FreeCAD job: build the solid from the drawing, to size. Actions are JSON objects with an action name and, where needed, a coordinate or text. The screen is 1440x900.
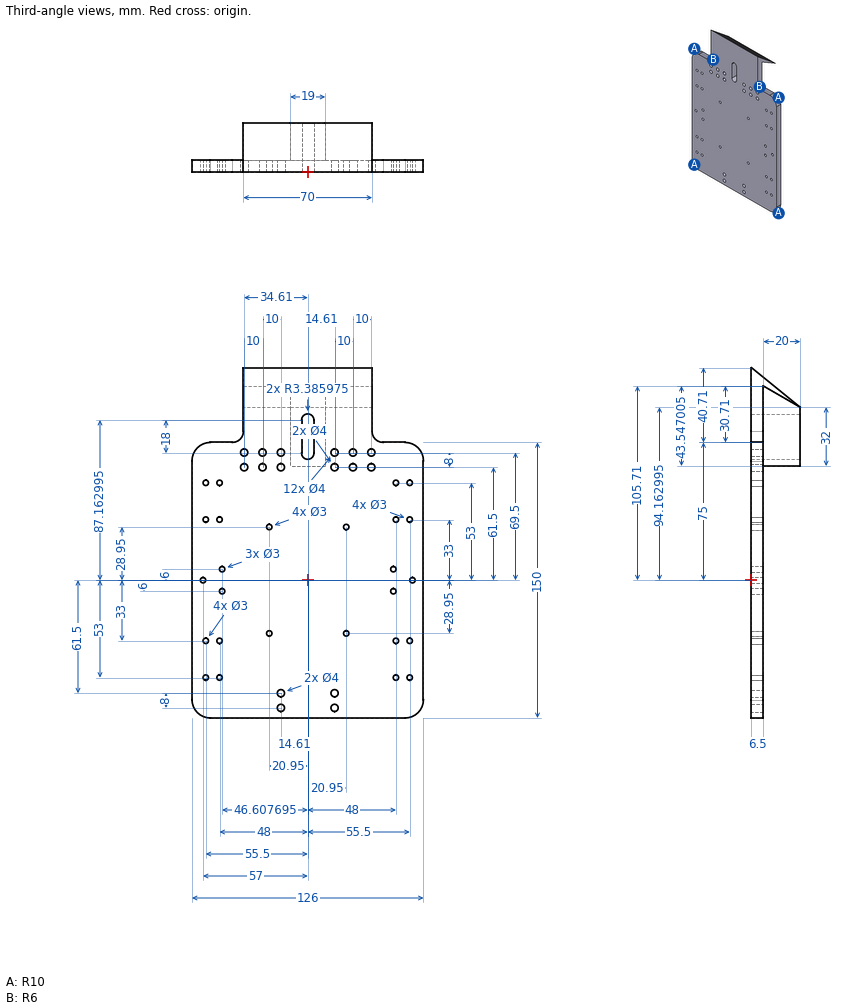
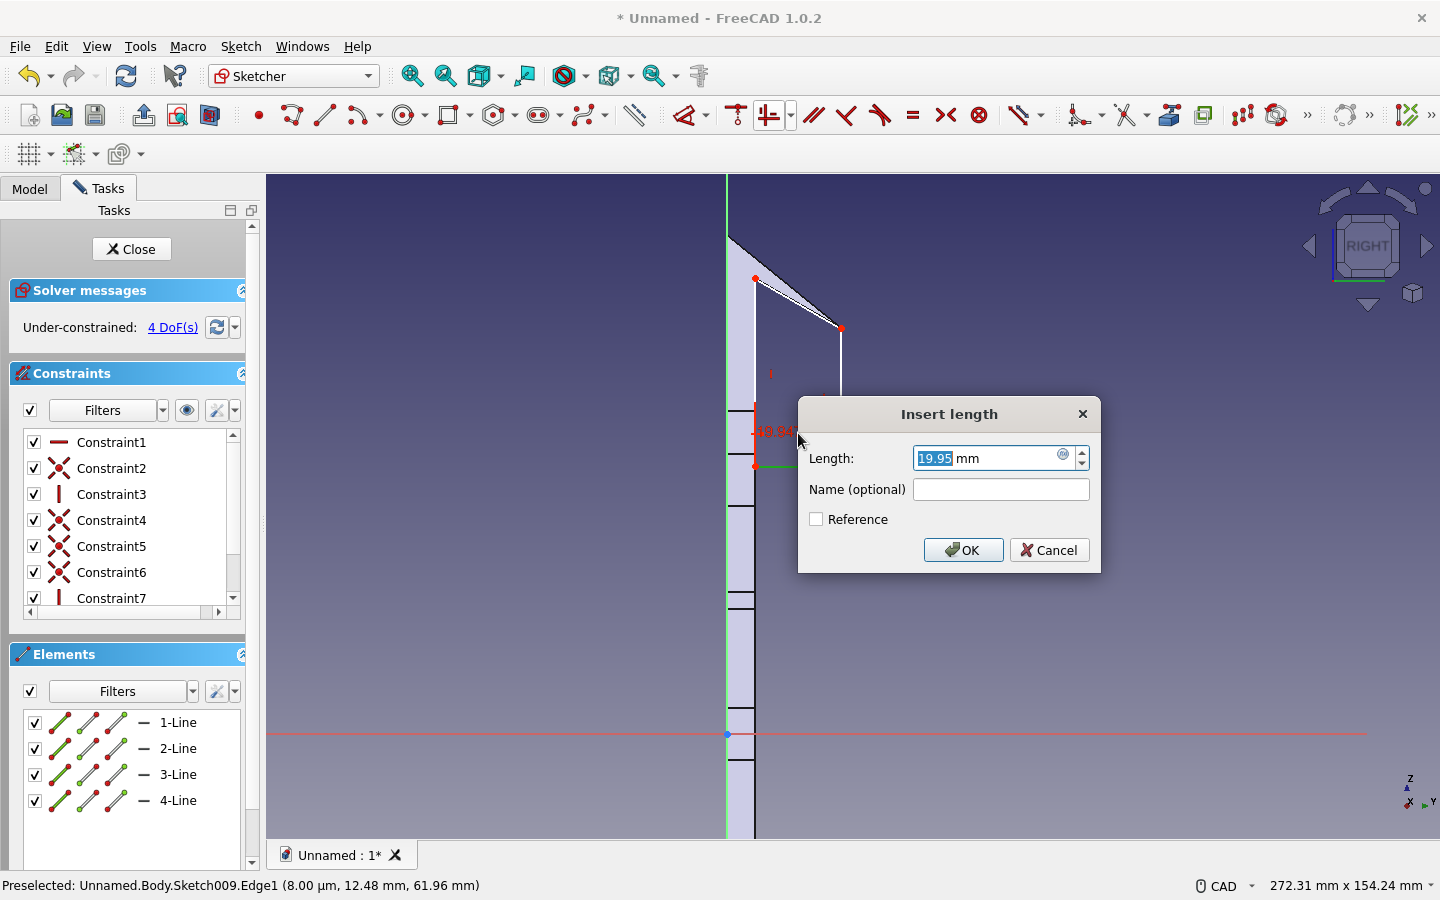
{"action": "type", "text": "20"}
{"action": "key", "text": "Return"}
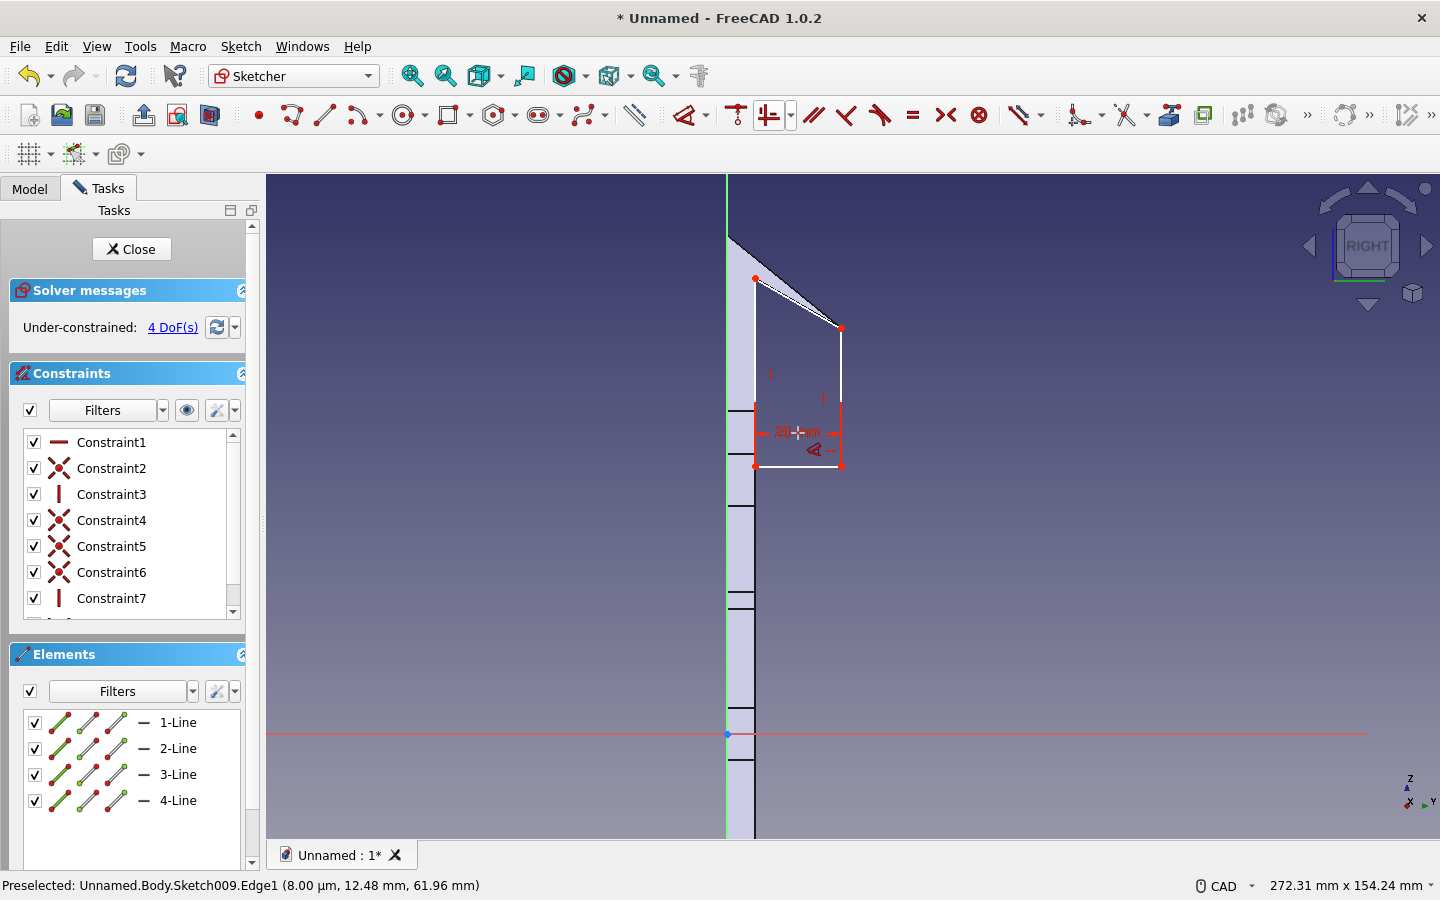
{"action": "left_click", "coordinate": [841, 426]}
{"action": "left_click", "coordinate": [875, 398]}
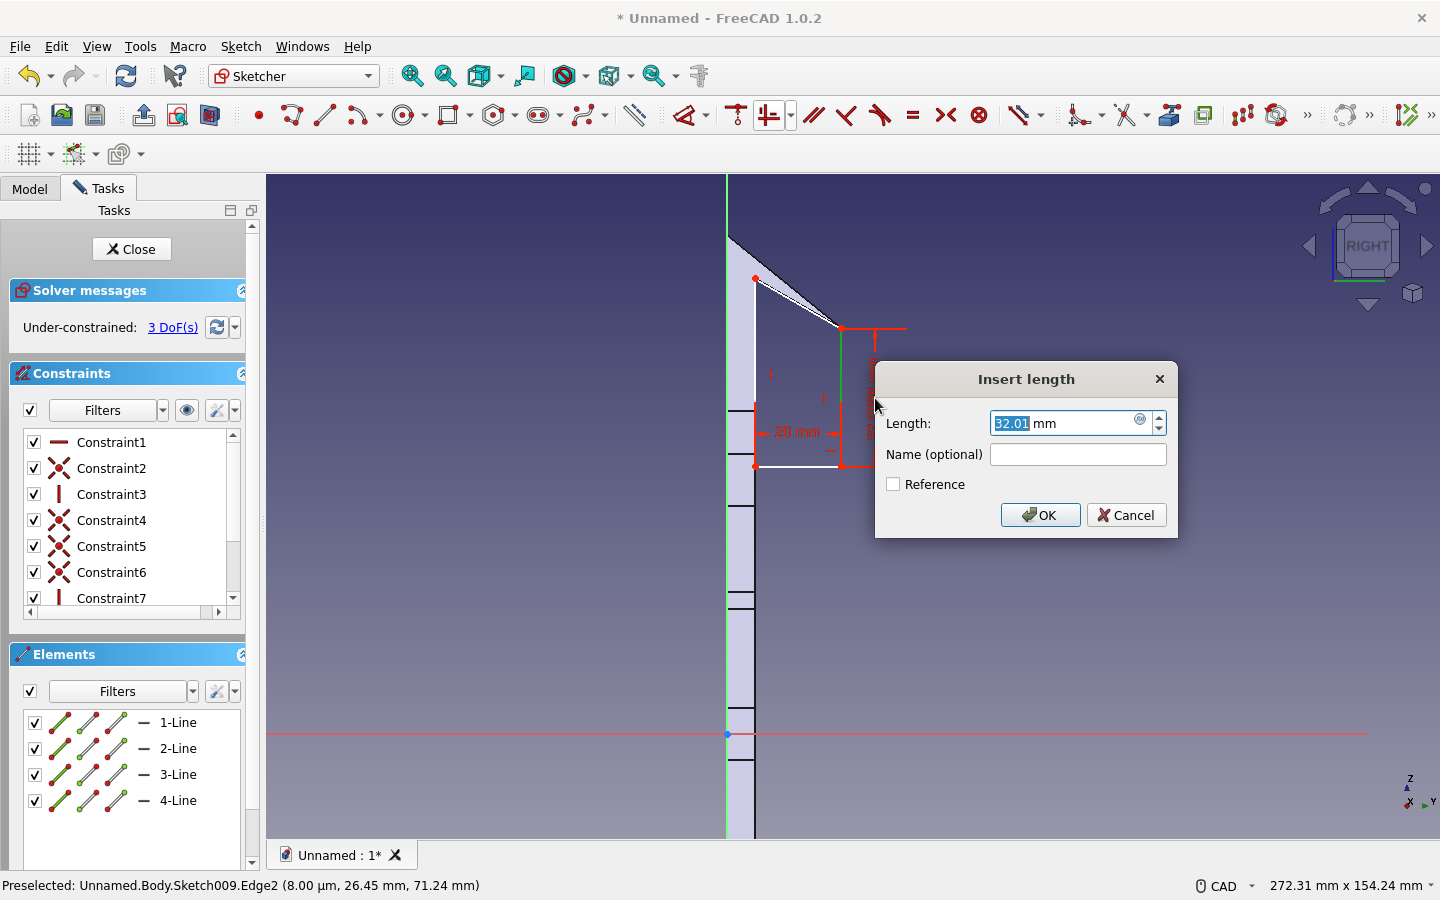
{"action": "type", "text": "32"}
{"action": "key", "text": "Return"}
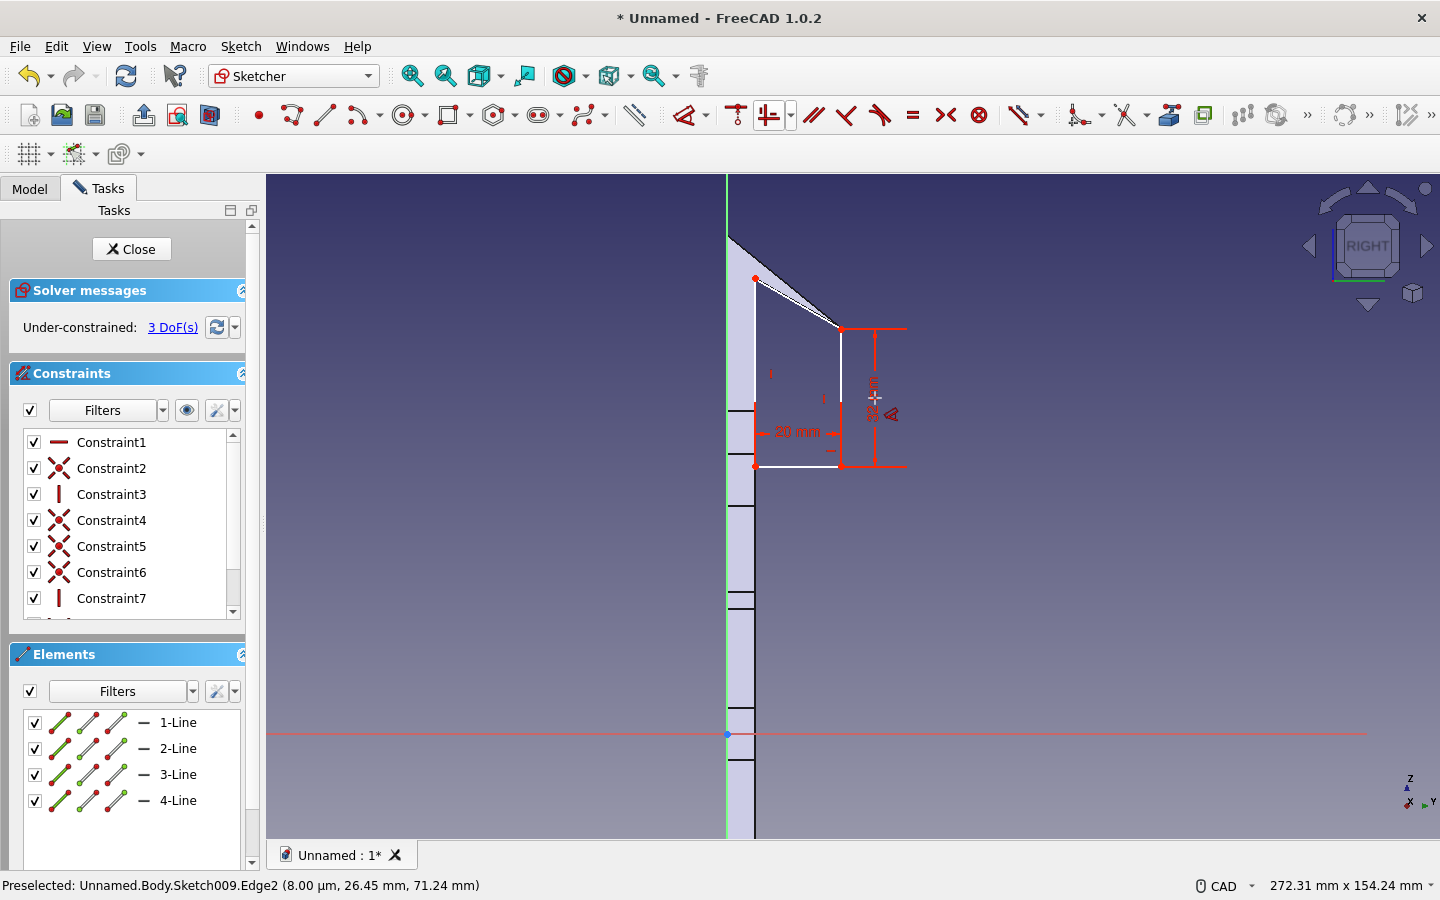
{"action": "scroll", "coordinate": [755, 467], "scroll_direction": "up", "scroll_amount": 2}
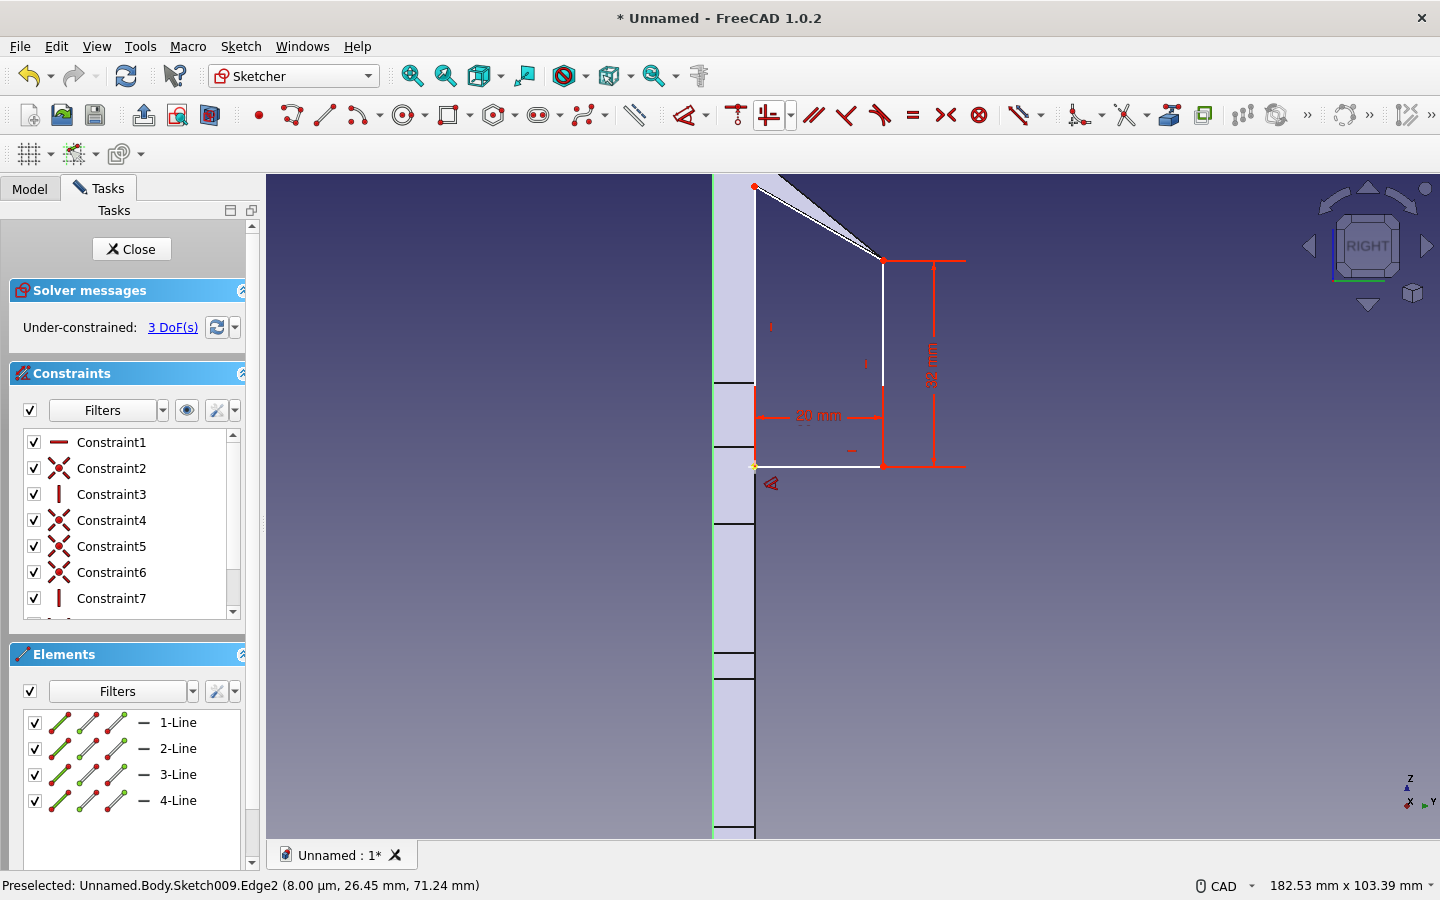
{"action": "left_click", "coordinate": [755, 467]}
{"action": "left_click", "coordinate": [734, 433]}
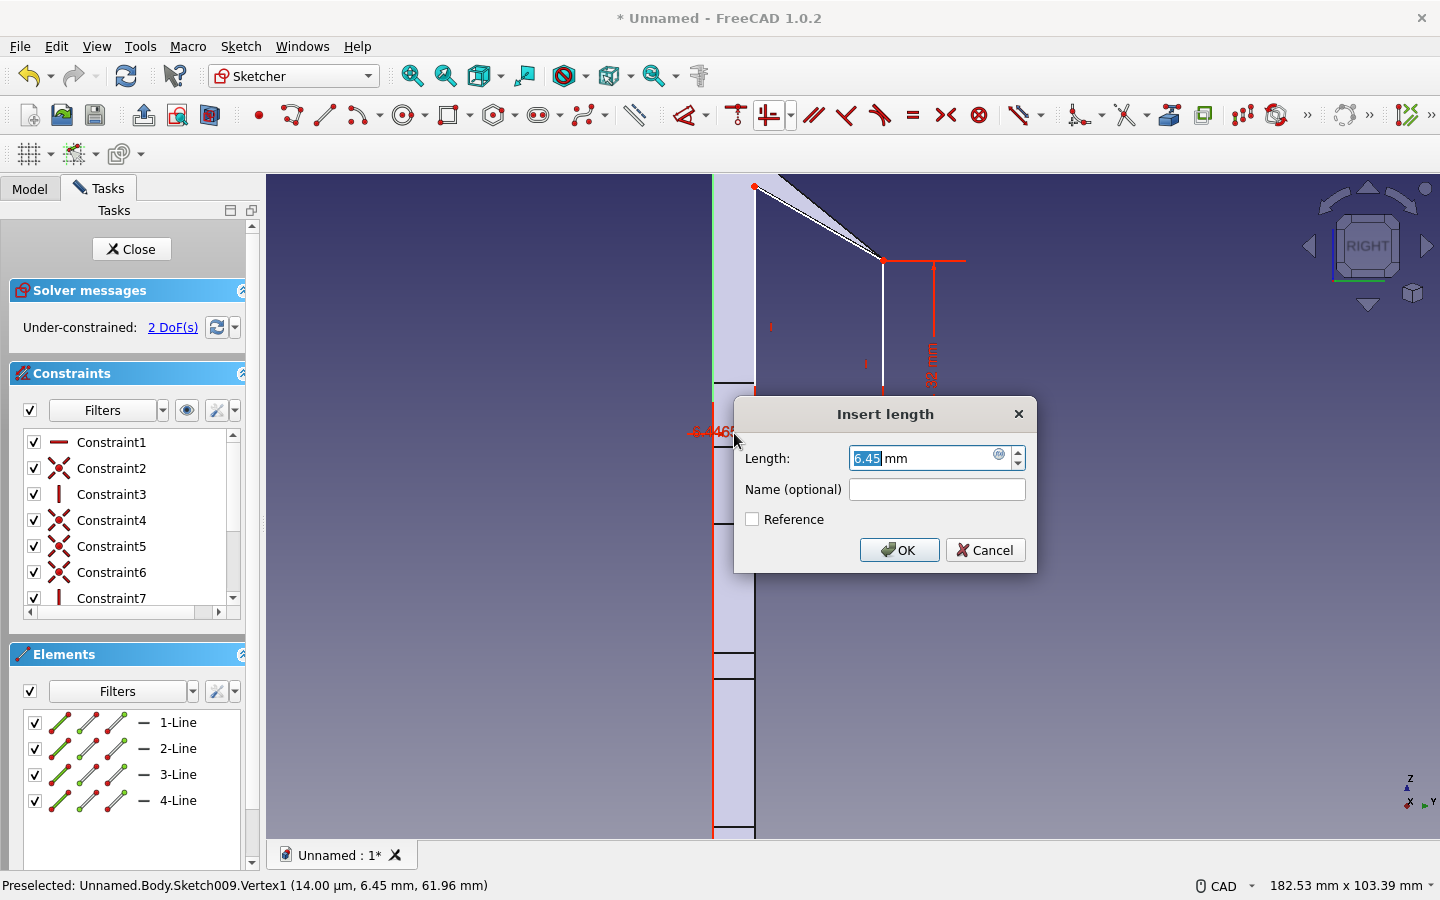
{"action": "type", "text": "6.5"}
{"action": "key", "text": "Return"}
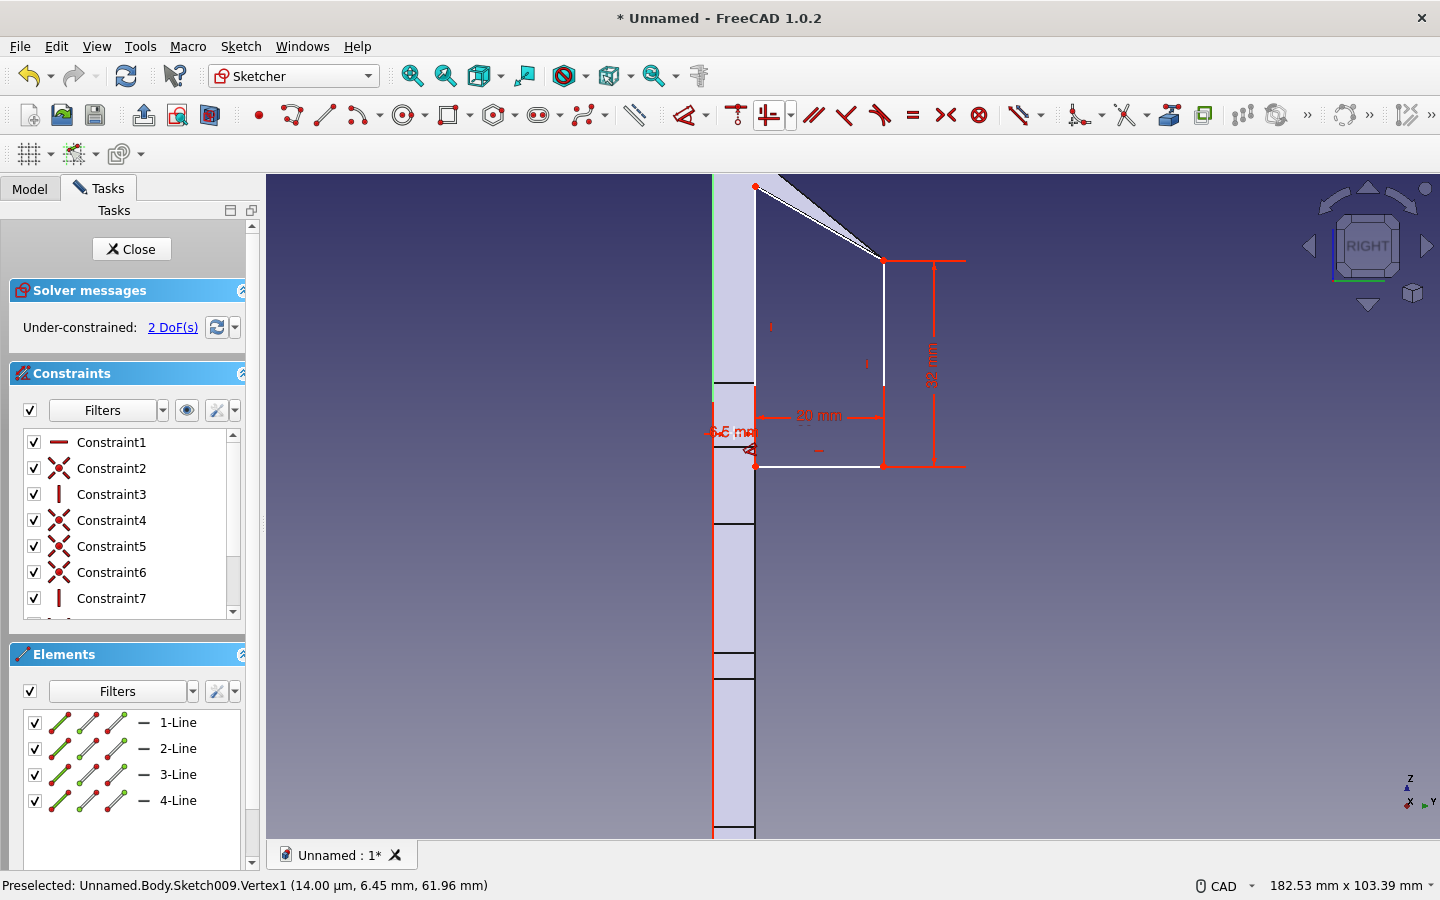
{"action": "scroll", "coordinate": [756, 468], "scroll_direction": "down", "scroll_amount": 2}